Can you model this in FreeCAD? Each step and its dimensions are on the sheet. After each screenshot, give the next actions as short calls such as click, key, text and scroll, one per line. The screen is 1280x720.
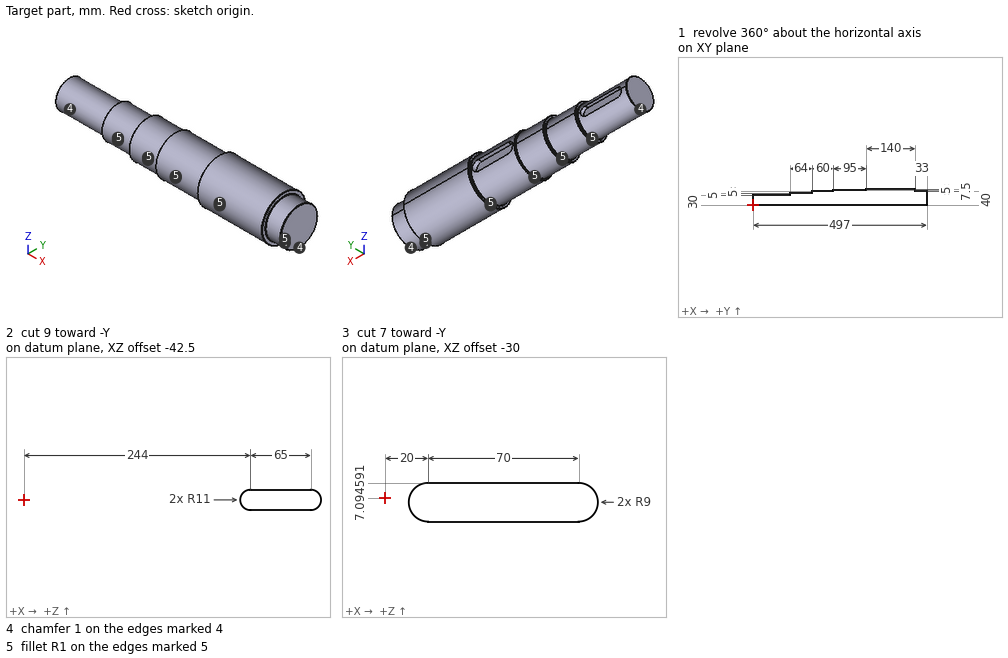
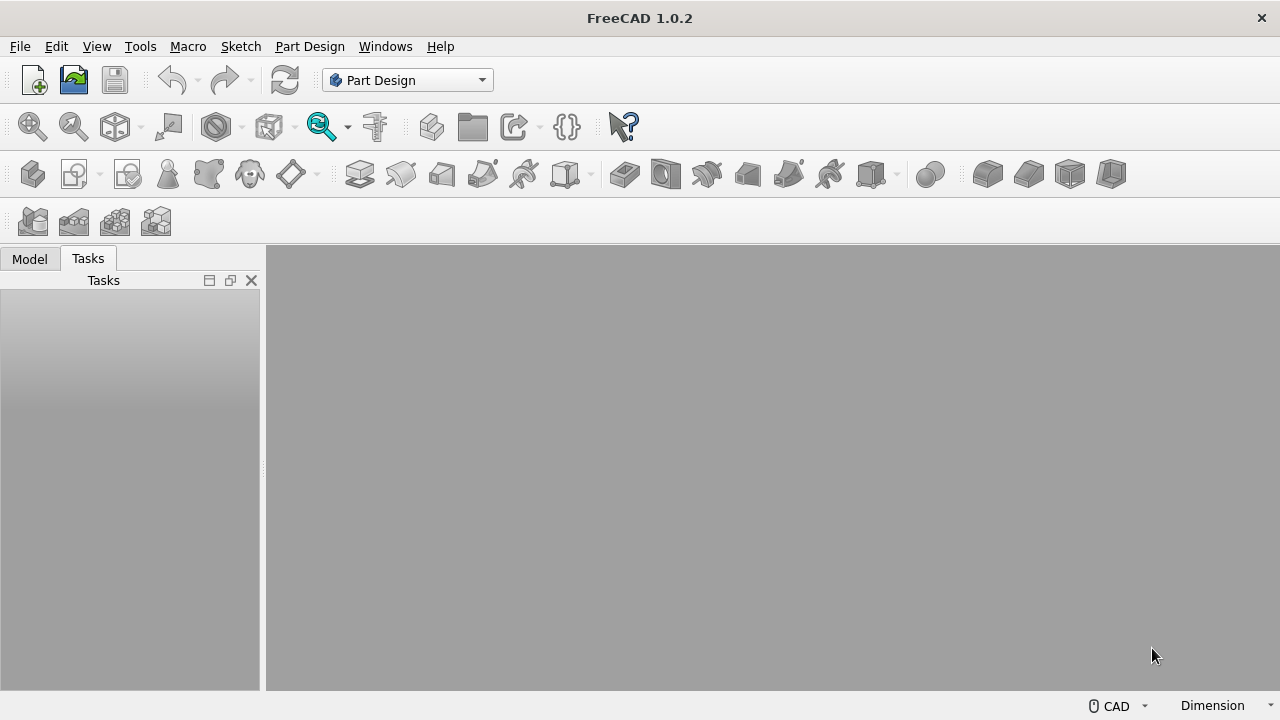
click(33, 80)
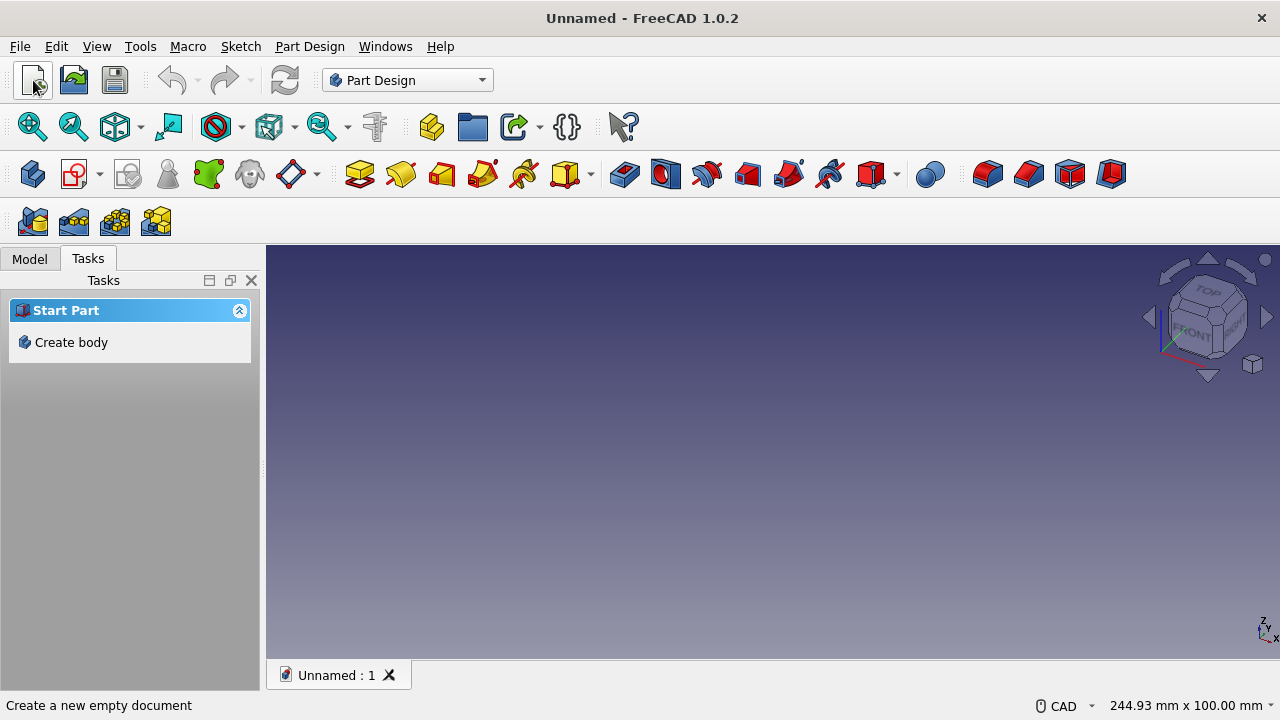
click(74, 174)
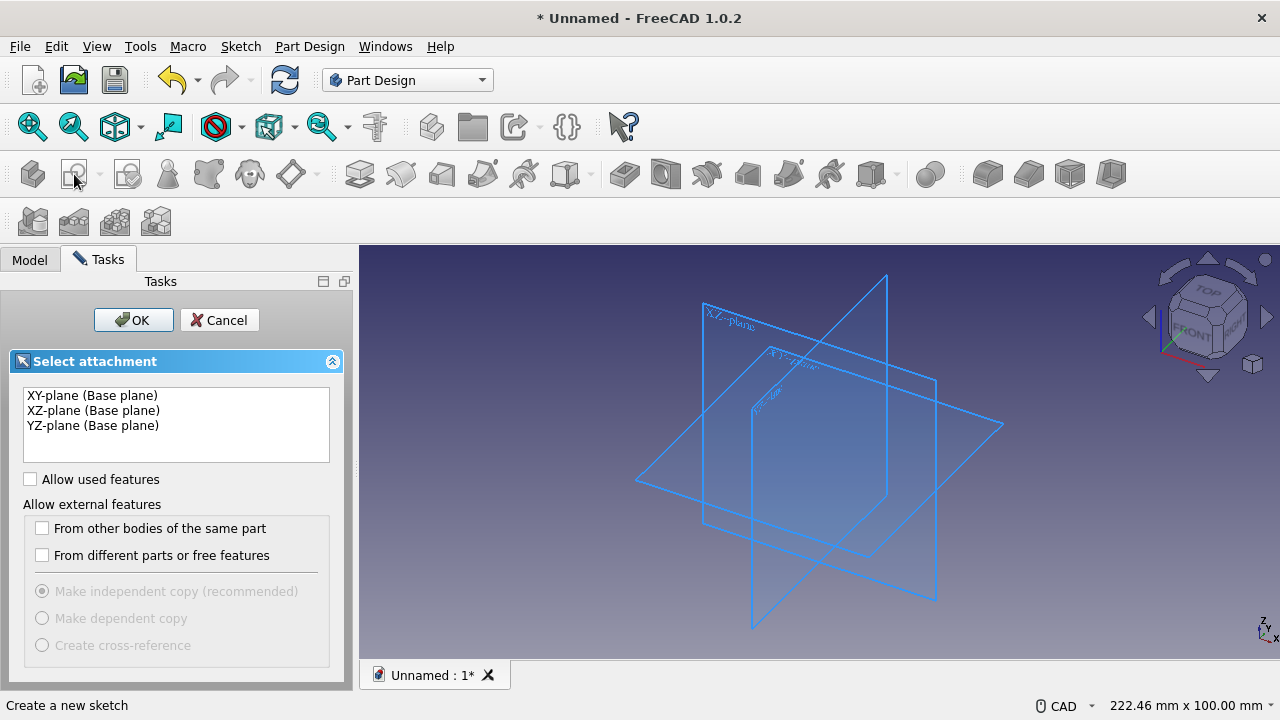
click(84, 396)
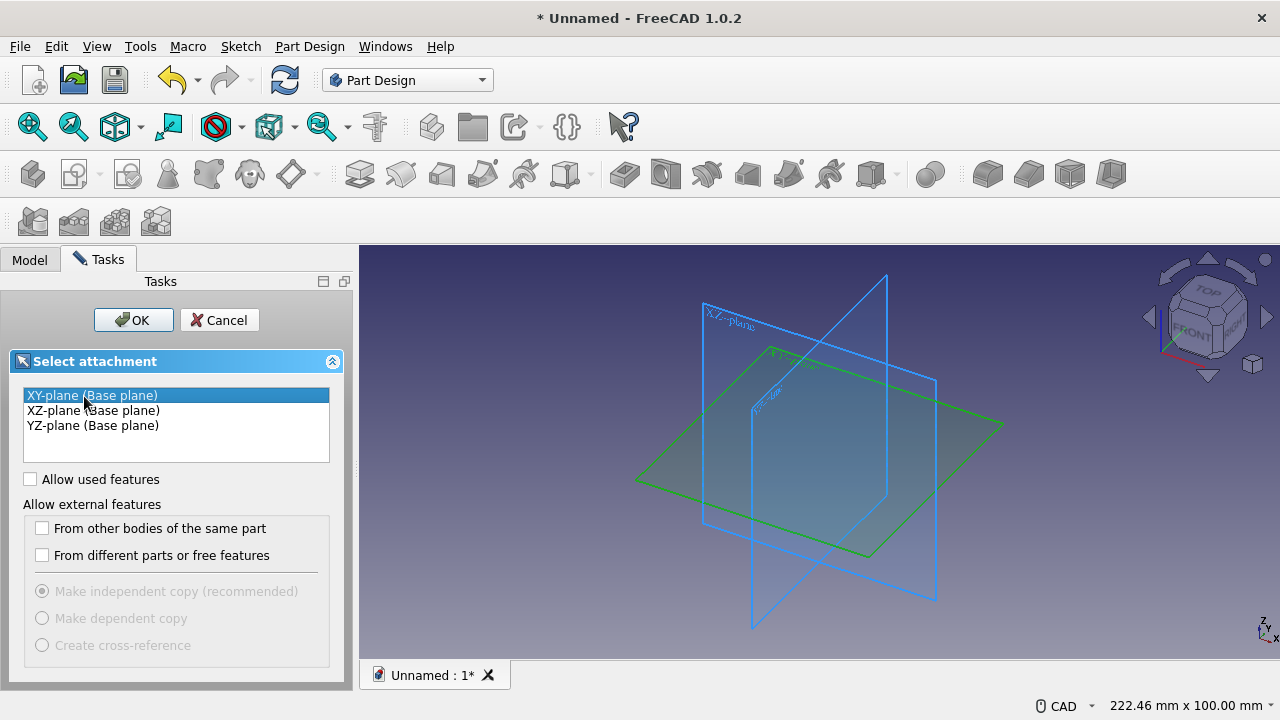
click(134, 320)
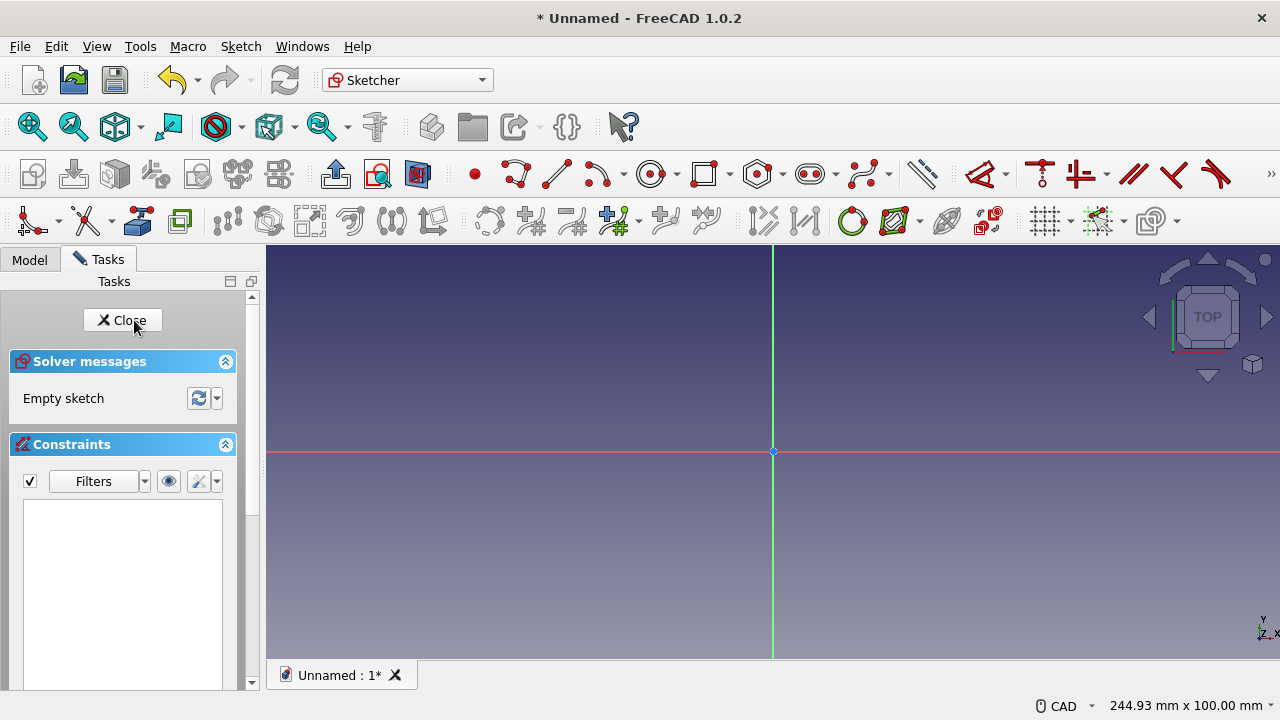
scroll(294, 494, down, 6)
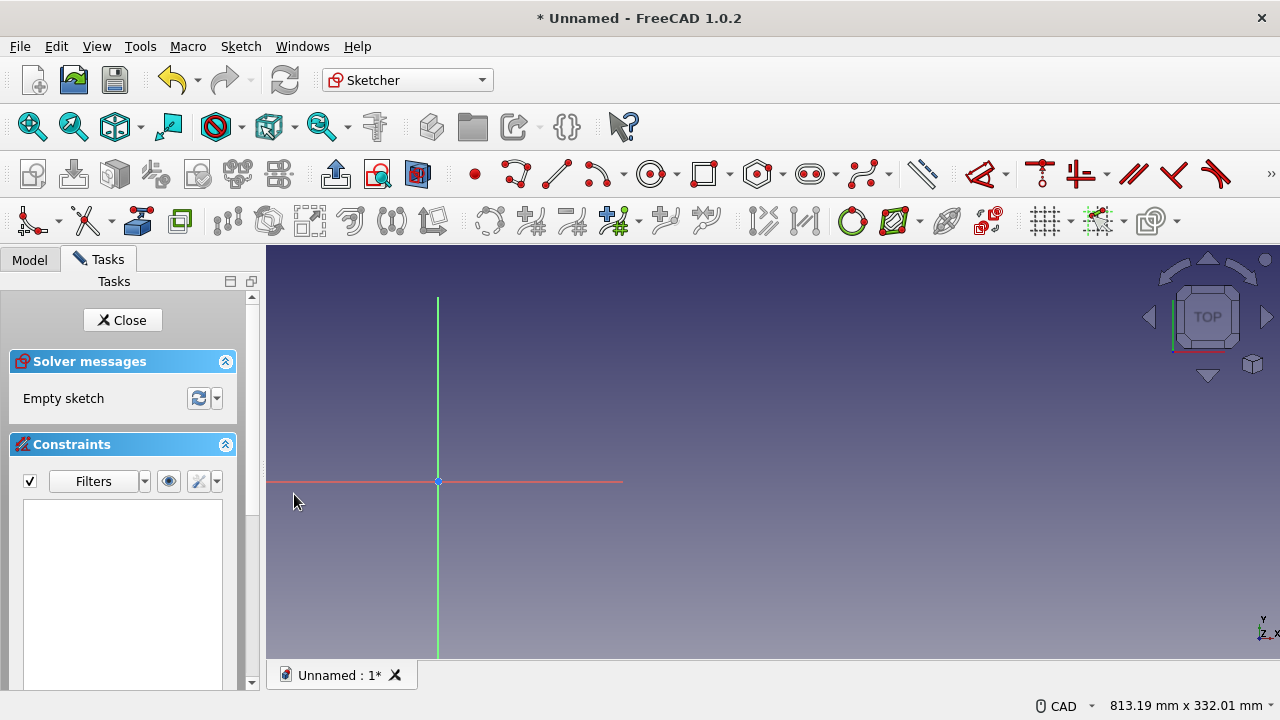
click(516, 174)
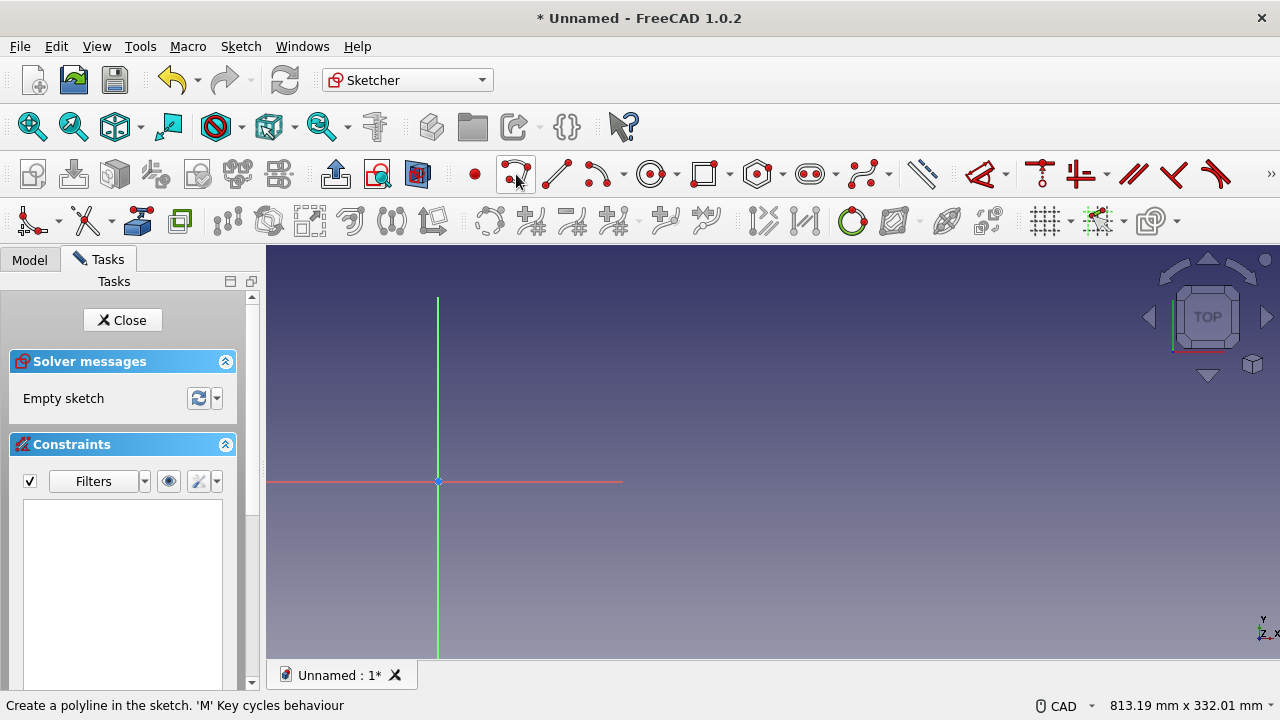
click(438, 482)
click(1058, 473)
click(1058, 432)
click(1017, 432)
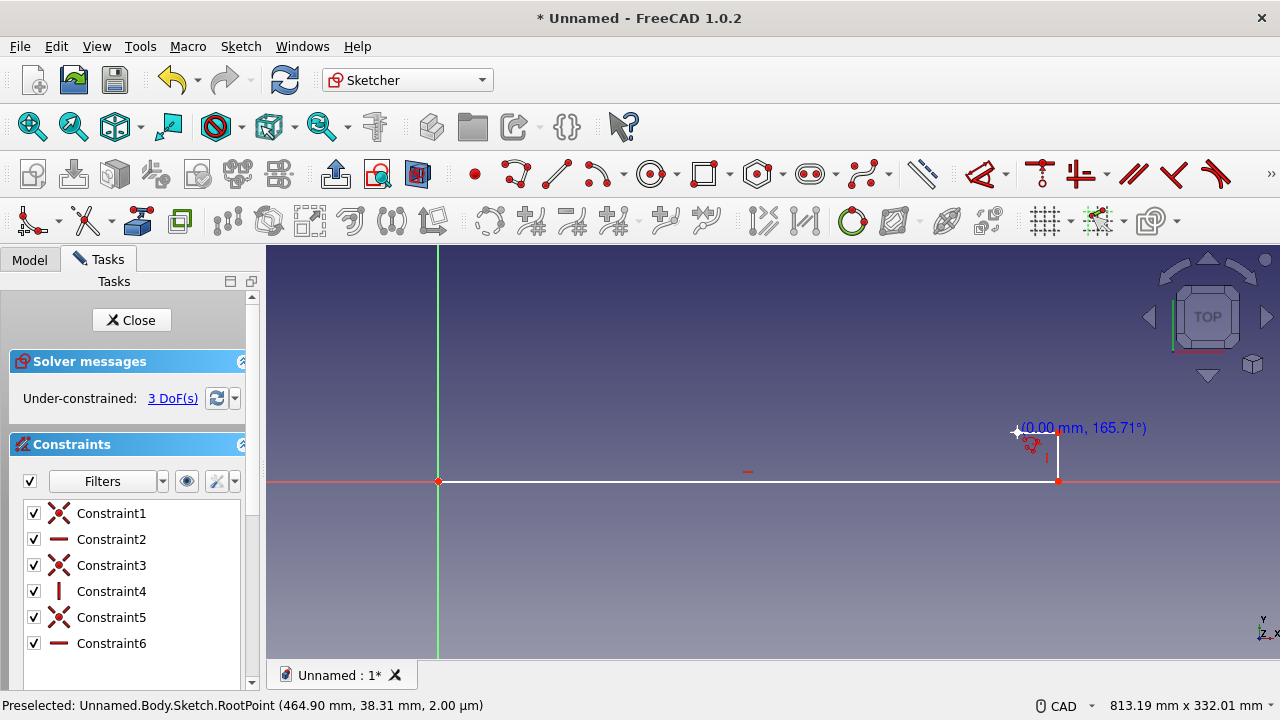
scroll(1017, 423, up, 3)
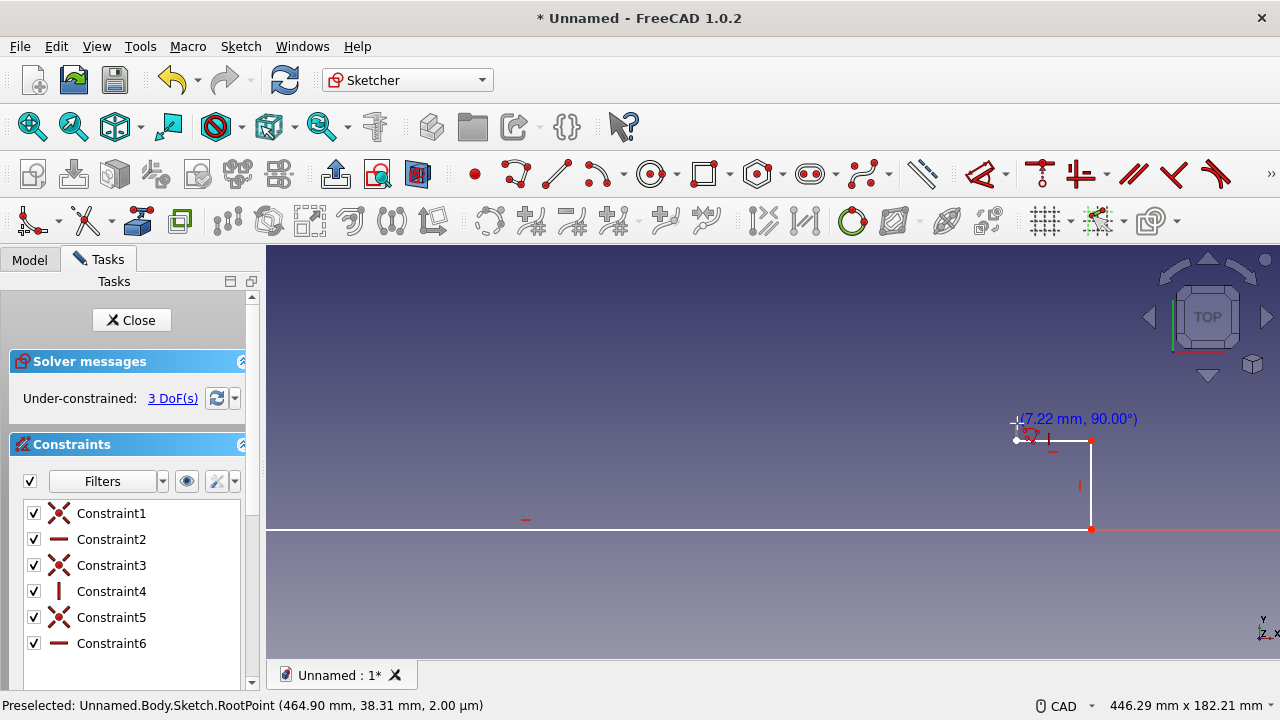
click(1016, 422)
click(698, 422)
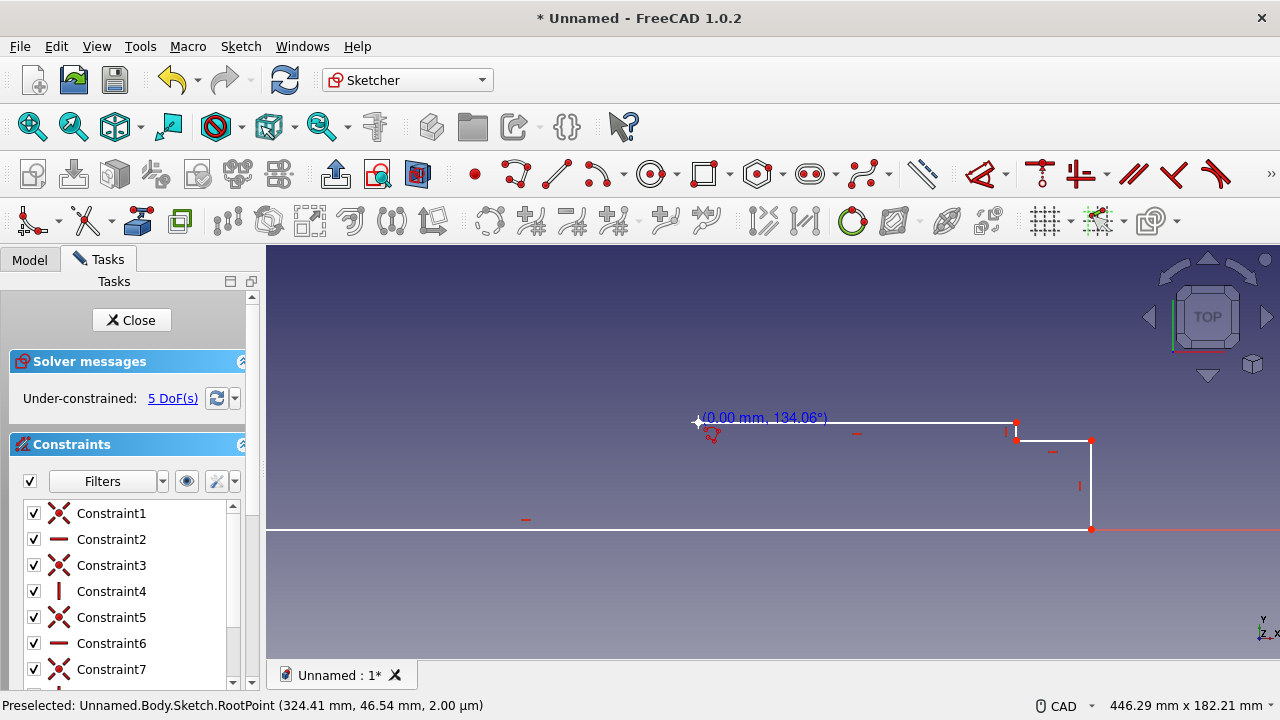
scroll(698, 433, up, 2)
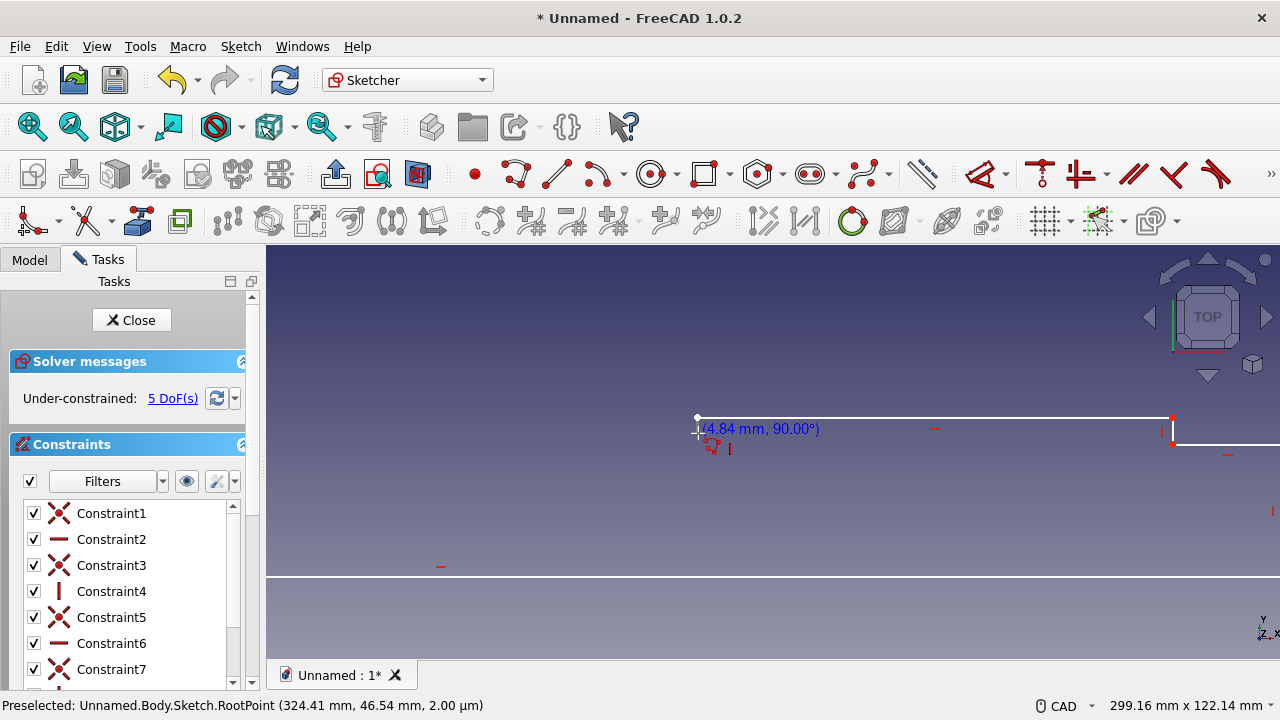
click(698, 433)
click(376, 433)